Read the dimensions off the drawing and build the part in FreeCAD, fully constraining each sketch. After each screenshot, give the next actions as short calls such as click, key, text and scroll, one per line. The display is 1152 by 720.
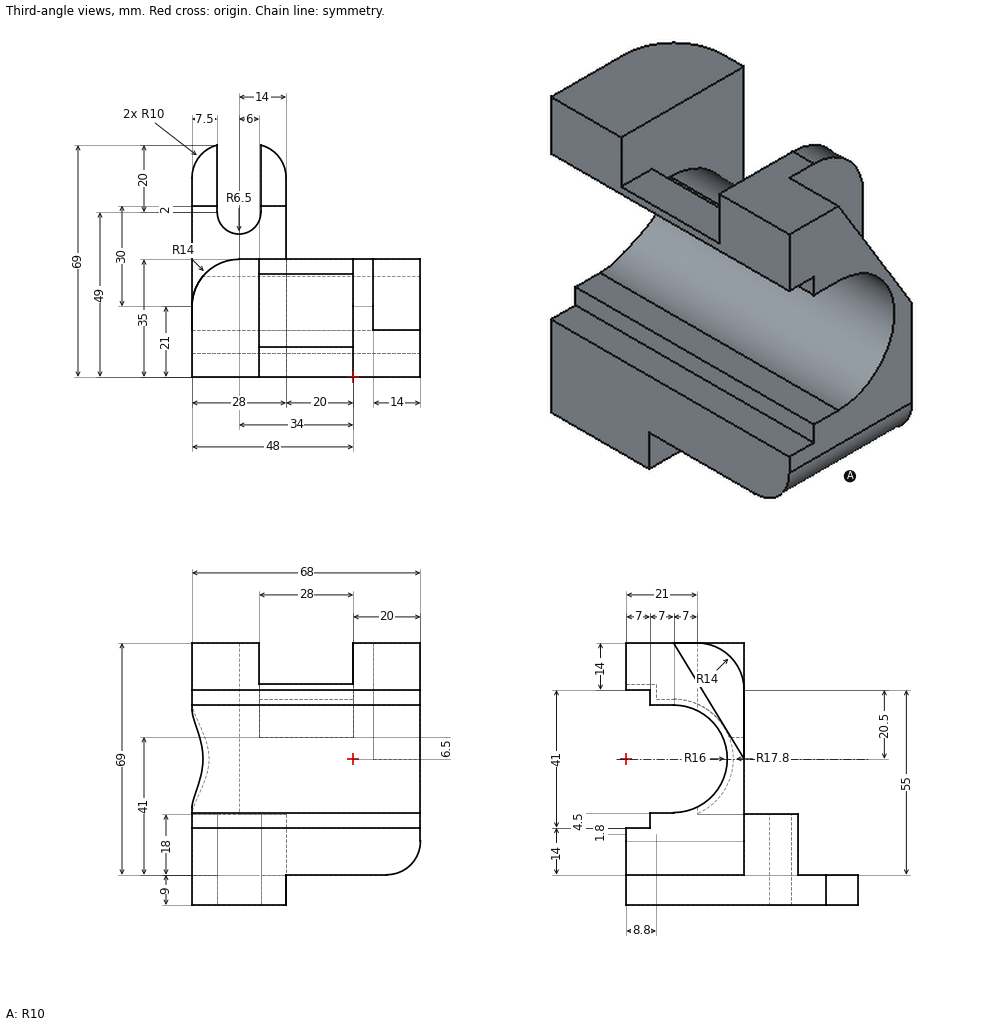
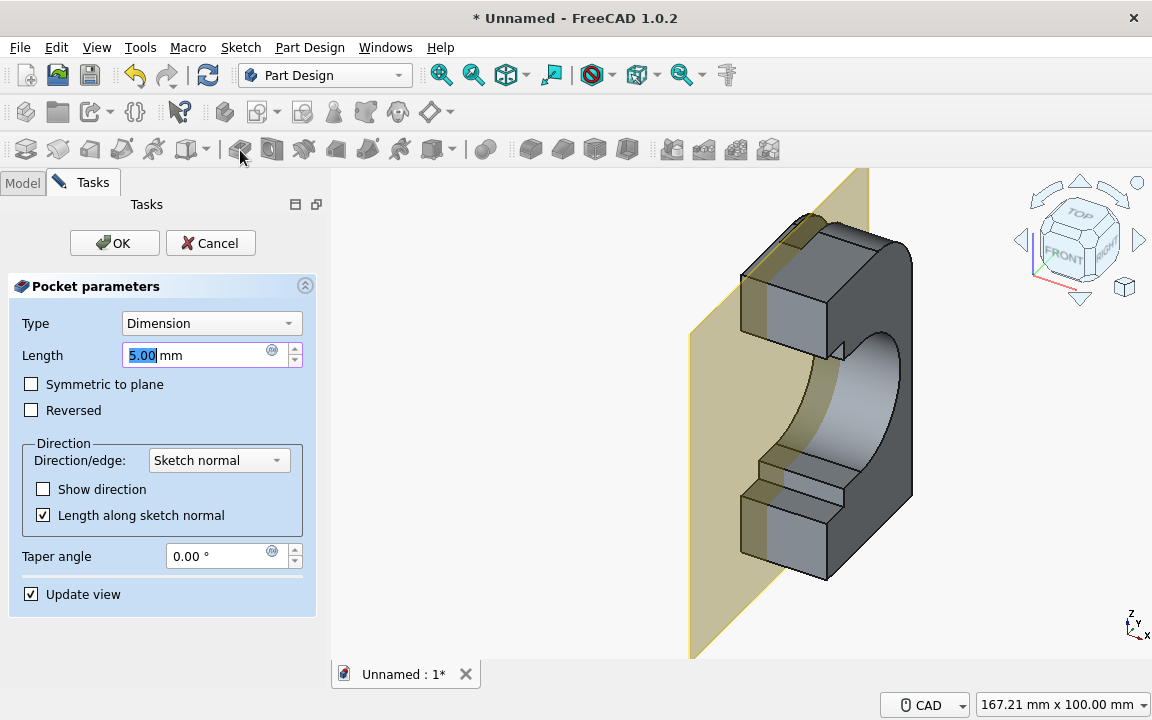
text(14)
key(Tab)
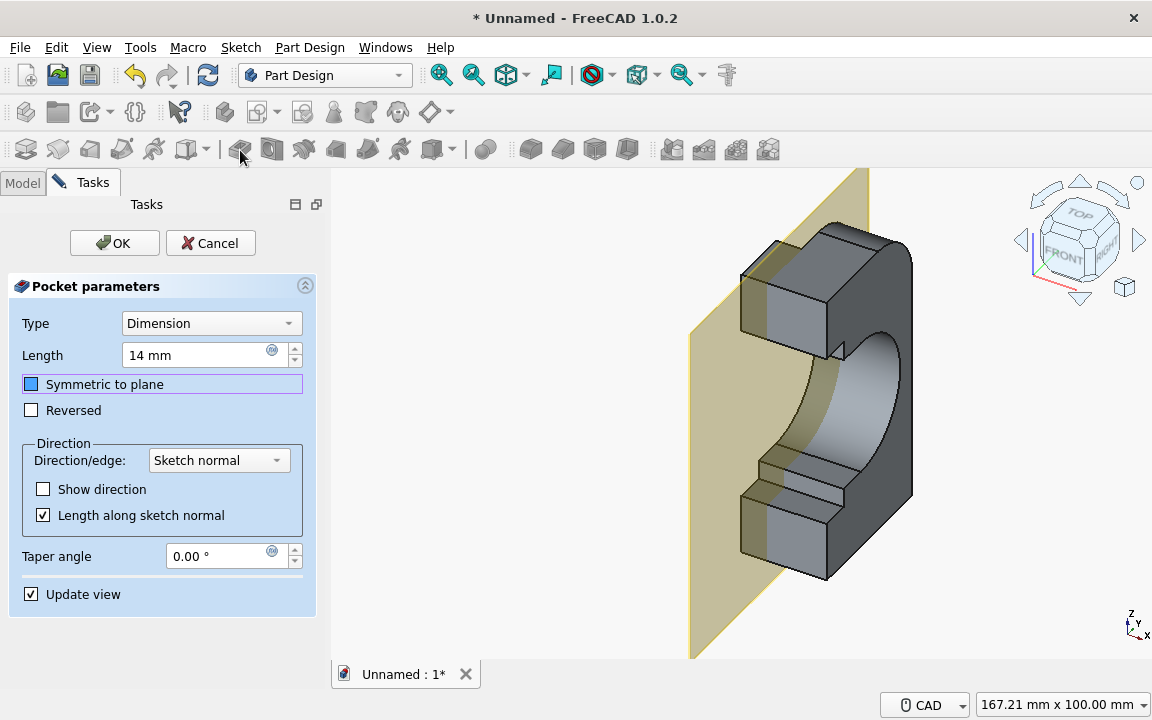
click(30, 410)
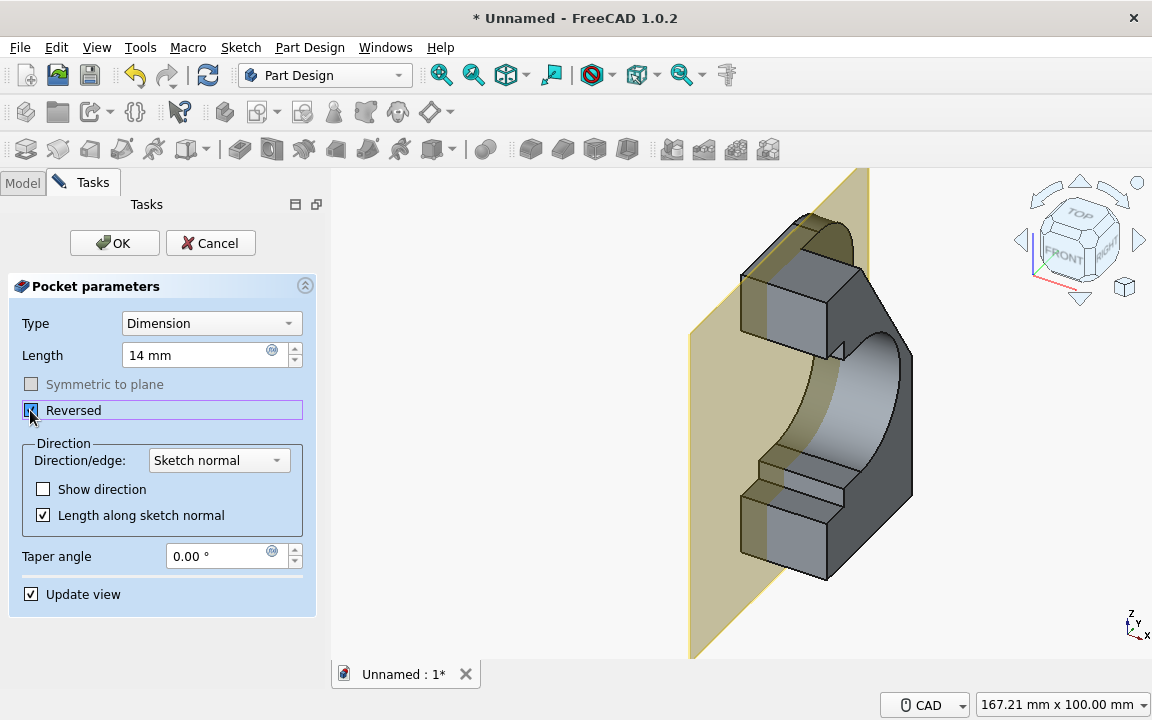
click(115, 243)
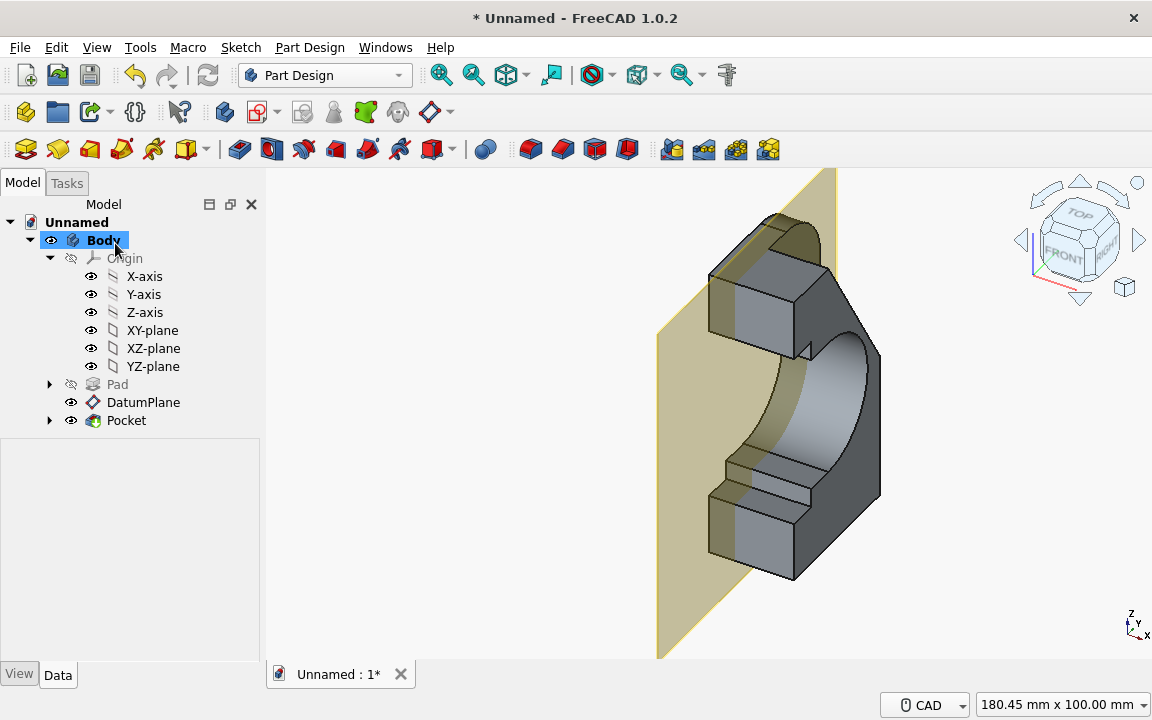
click(116, 402)
key(space)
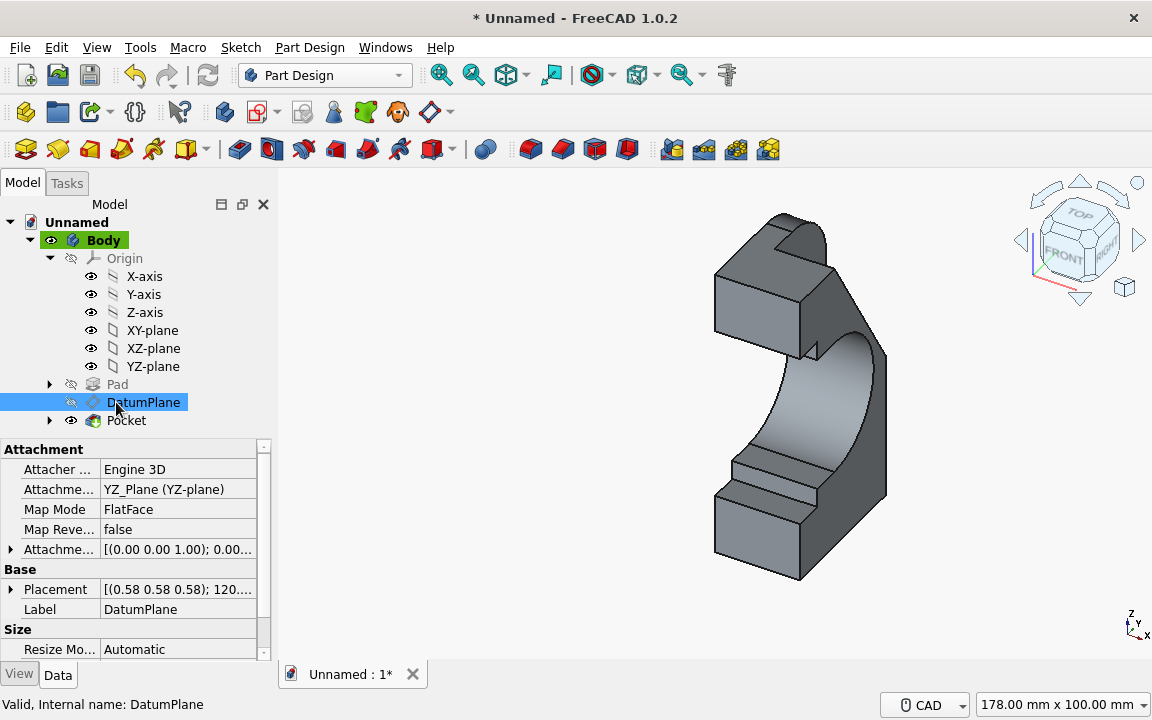
click(136, 366)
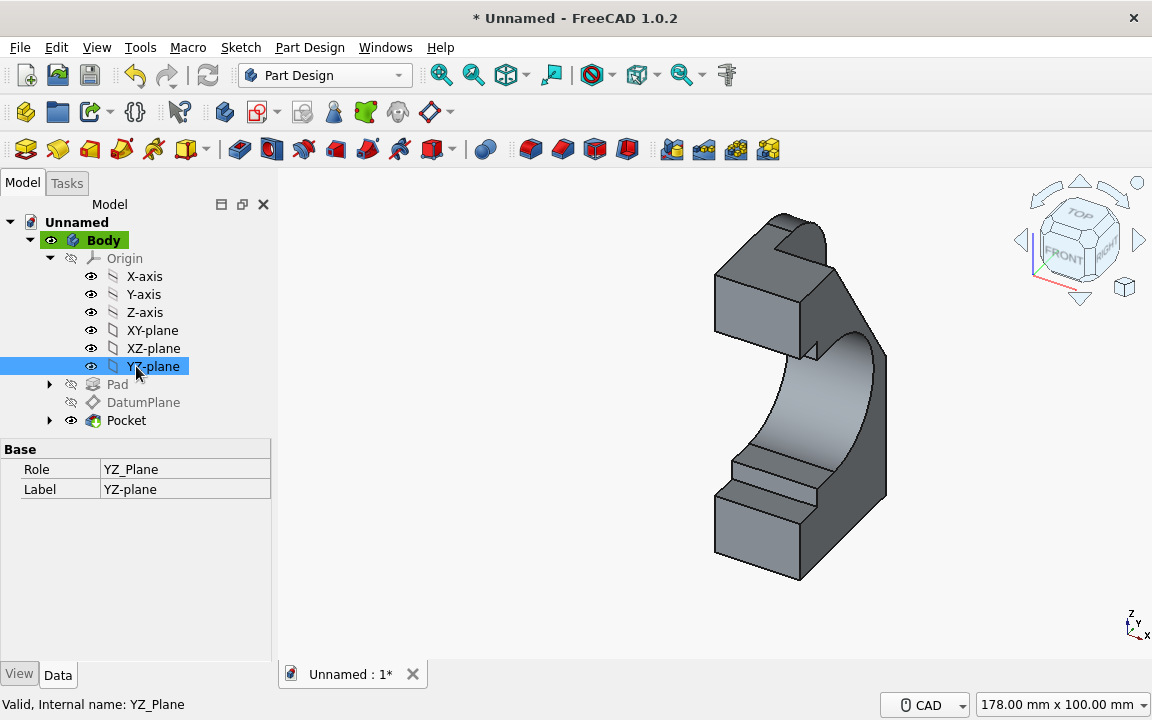
click(430, 112)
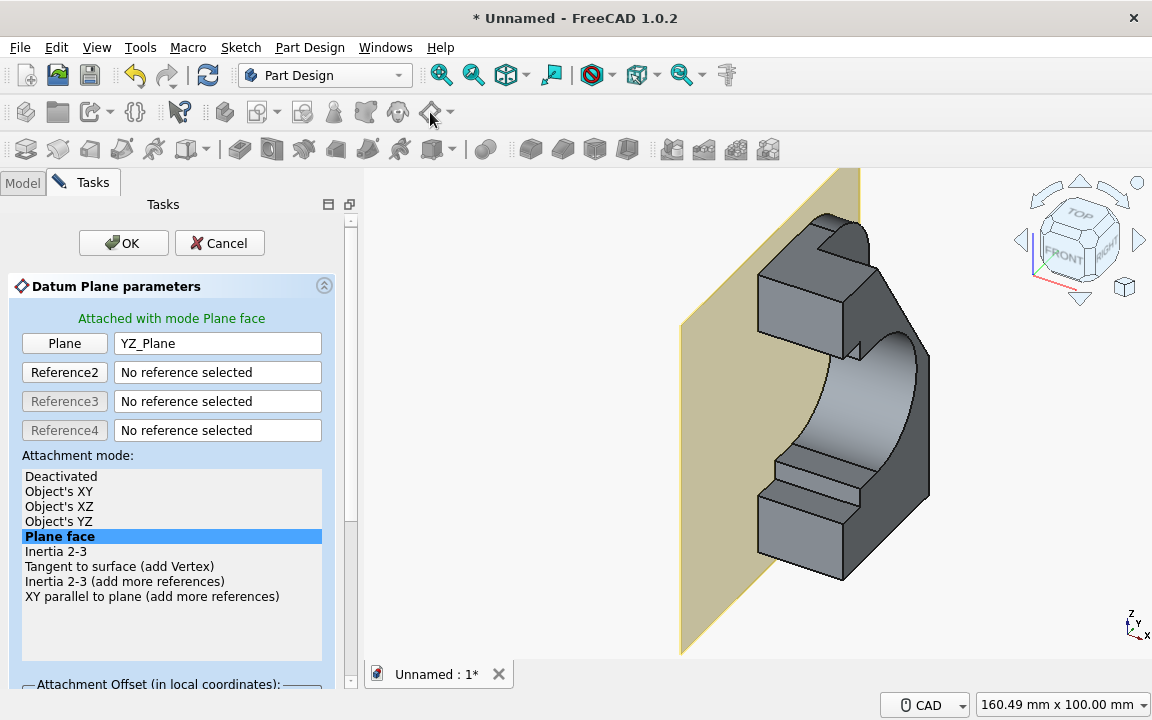
scroll(351, 451, down, 3)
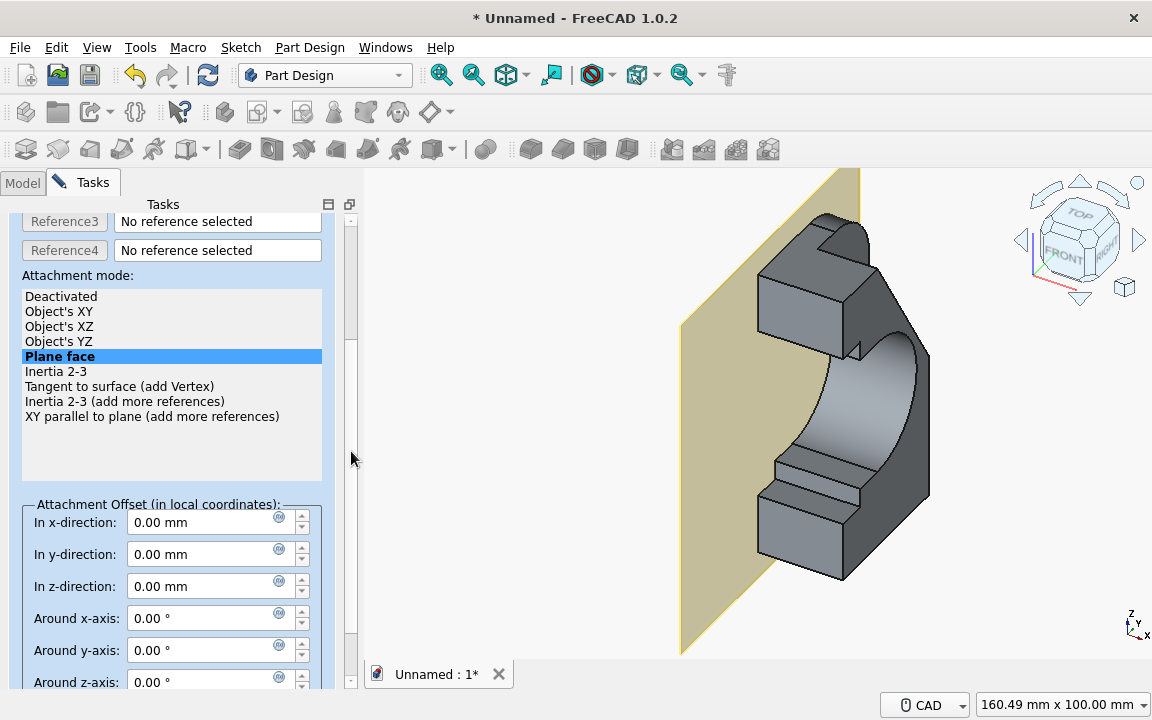
triple_click(210, 586)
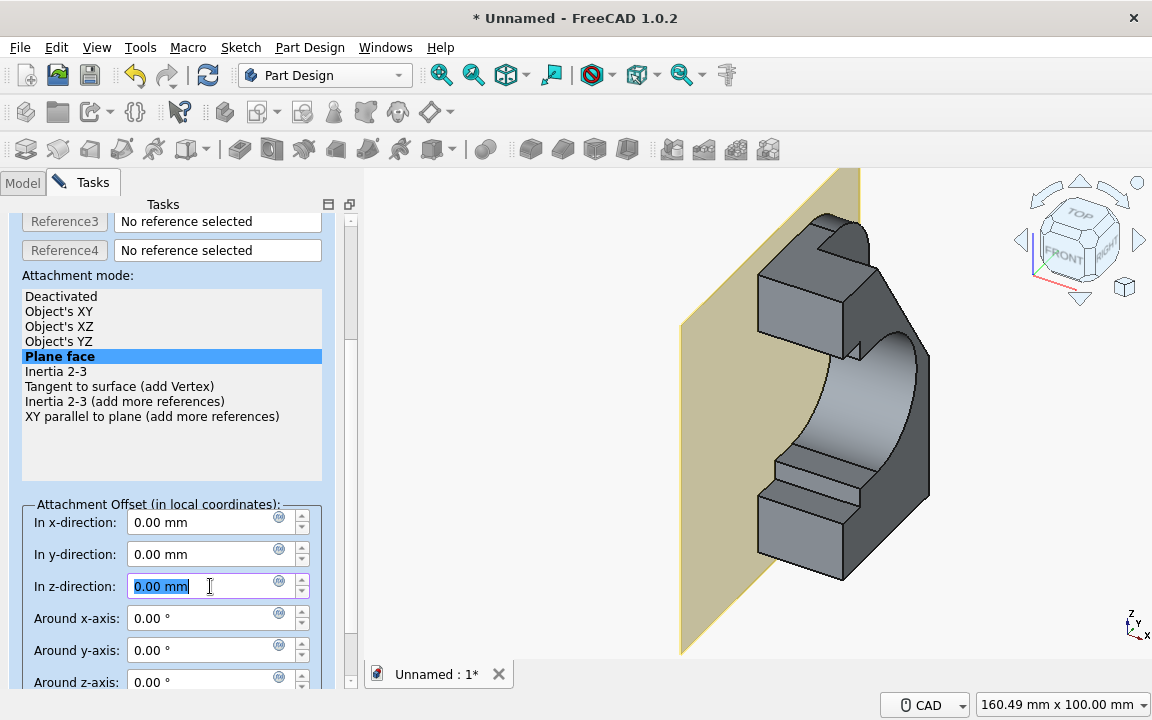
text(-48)
key(Tab)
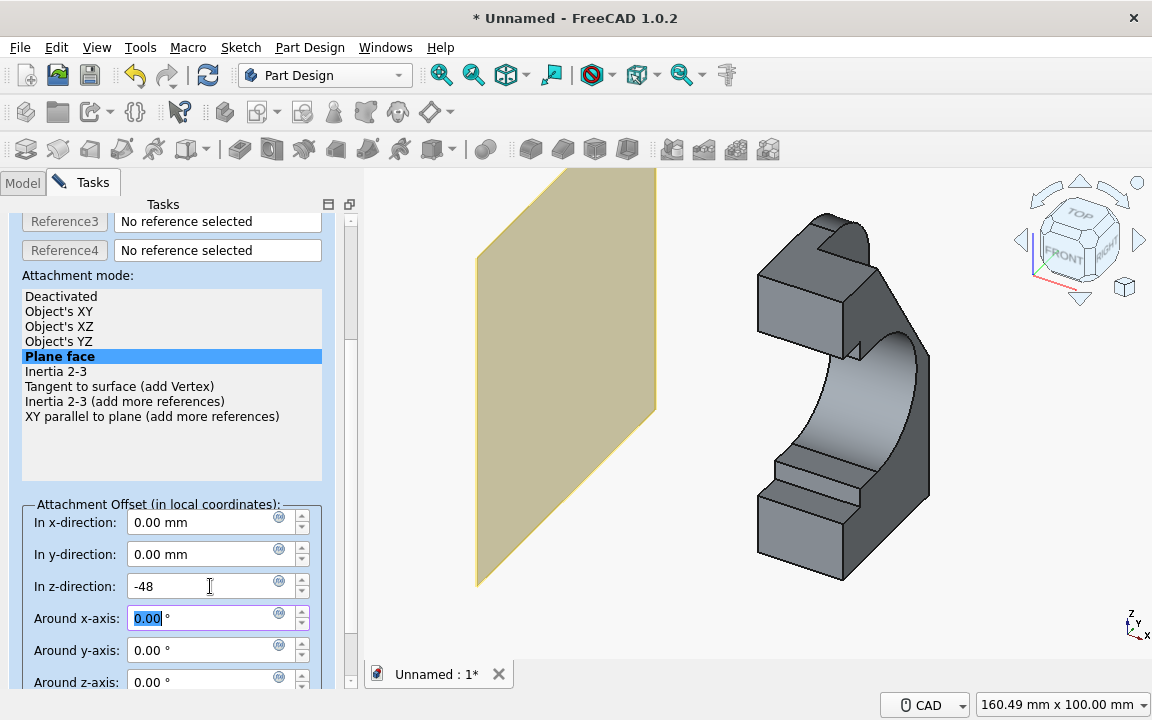
scroll(351, 451, up, 4)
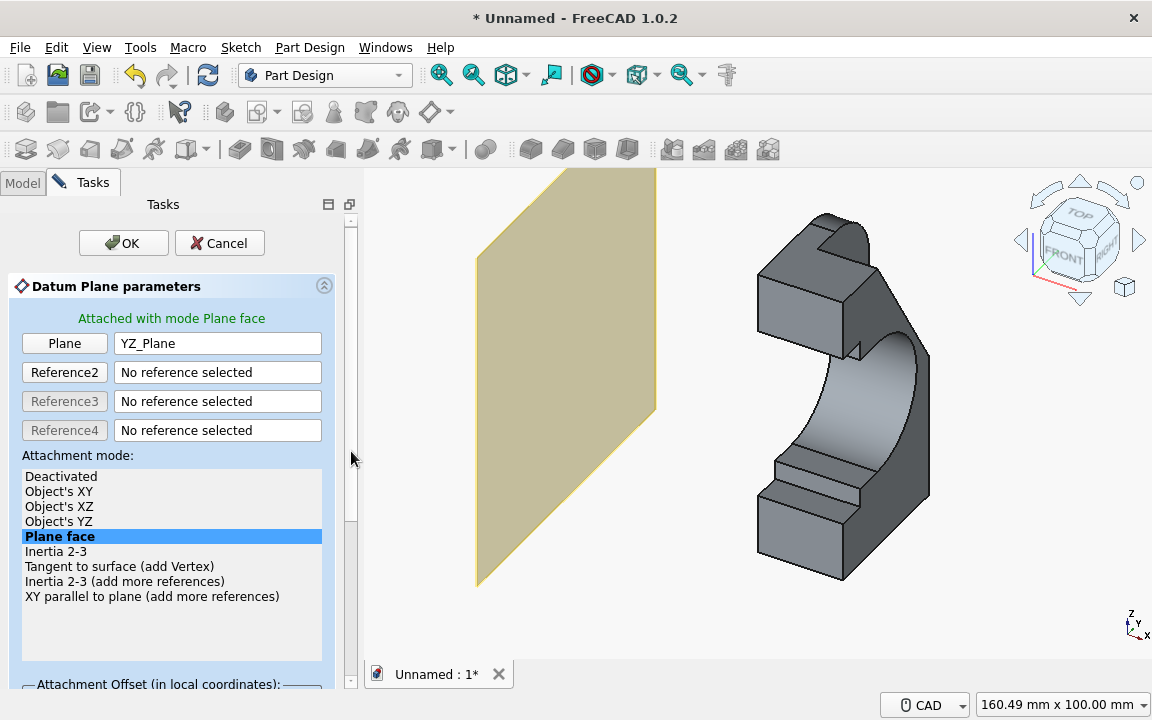
click(124, 243)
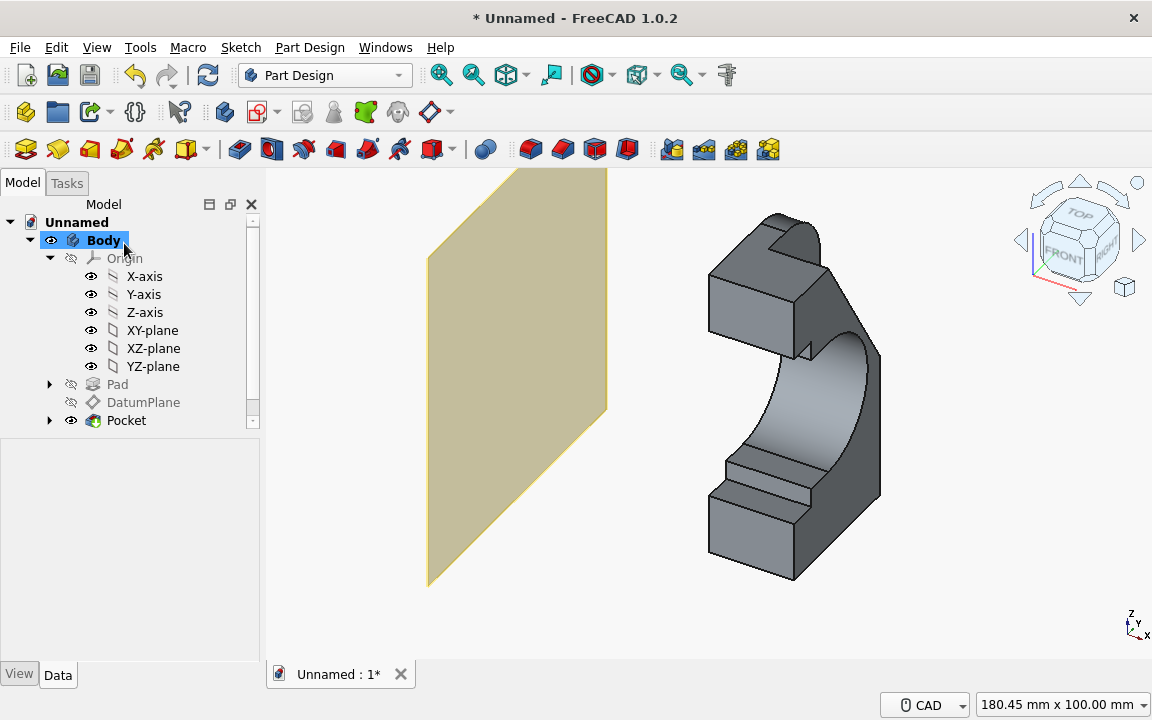
scroll(100, 326, down, 3)